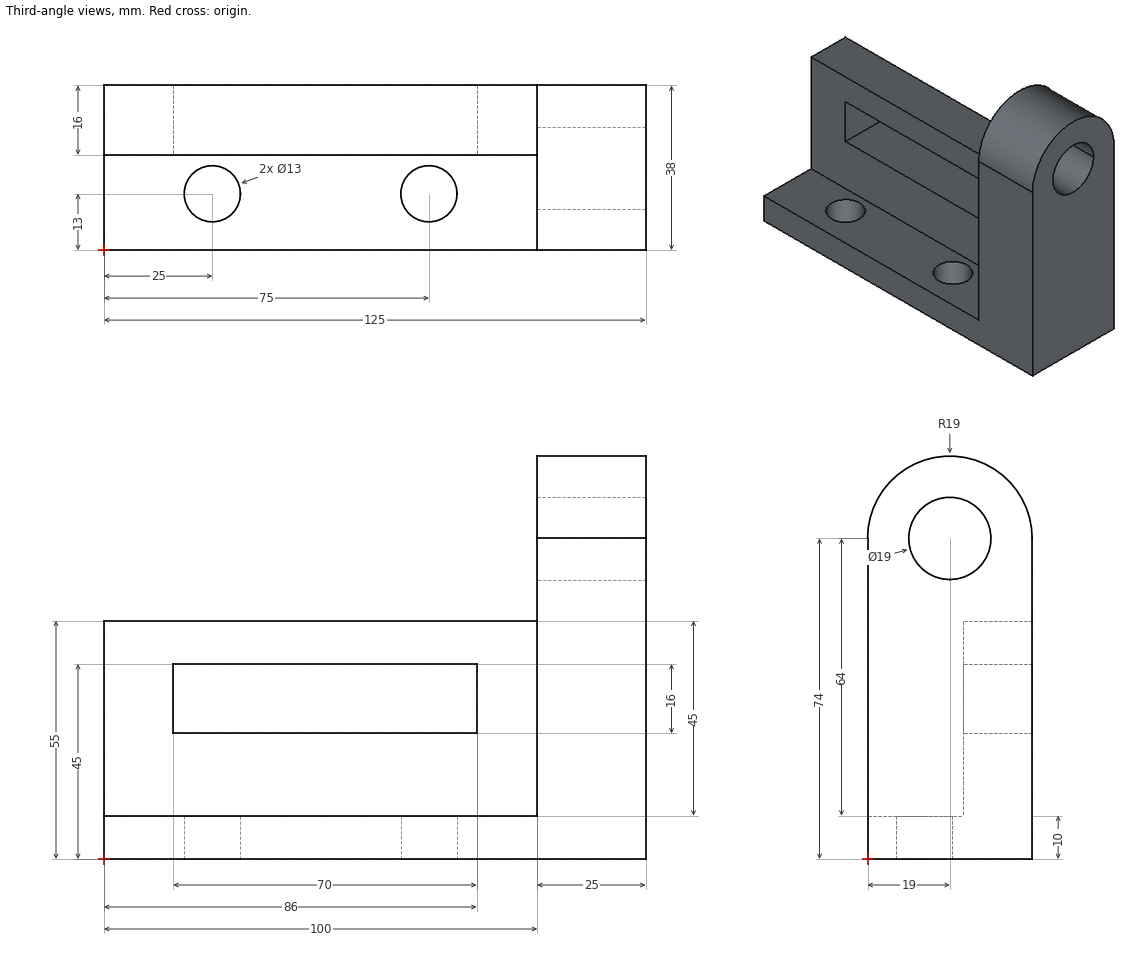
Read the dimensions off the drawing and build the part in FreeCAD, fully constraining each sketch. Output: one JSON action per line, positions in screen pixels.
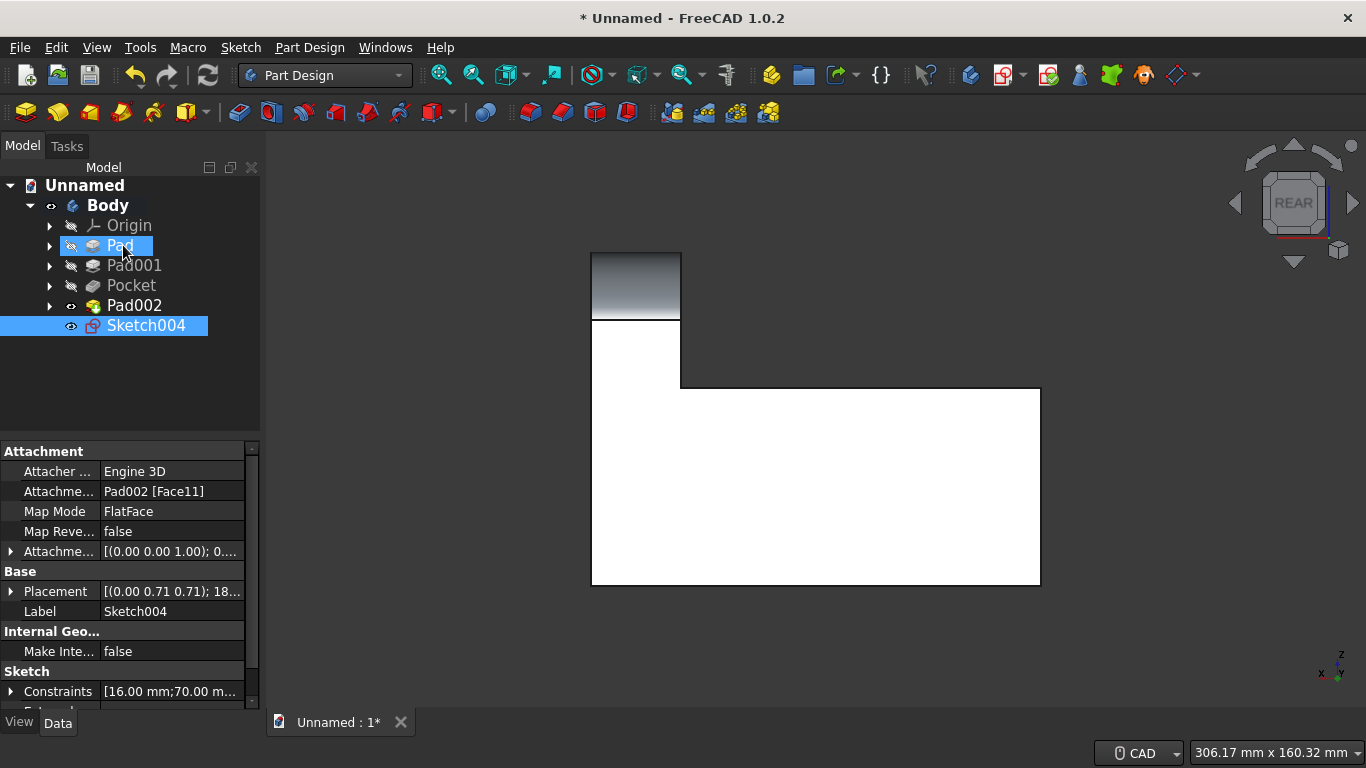
{"action": "left_click", "coordinate": [240, 112]}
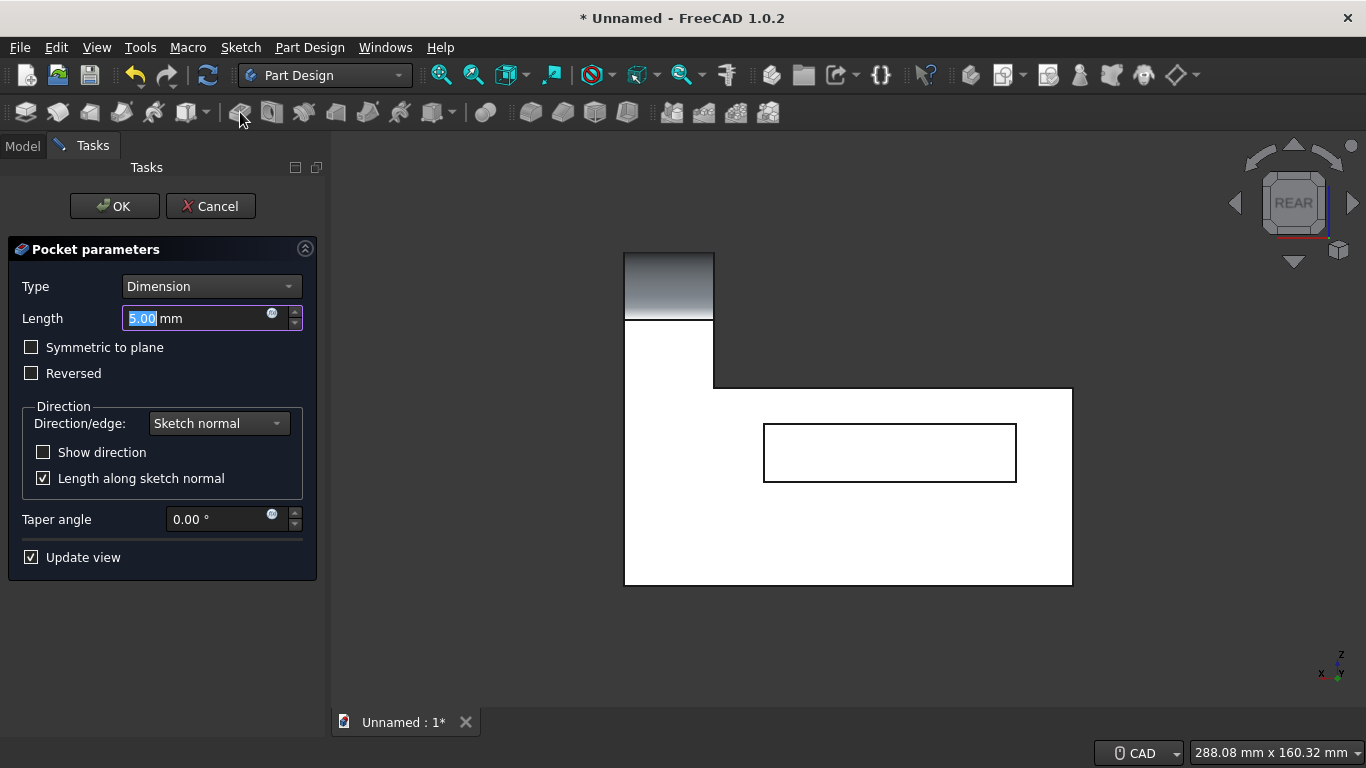
{"action": "type", "text": "16"}
{"action": "key", "text": "Tab"}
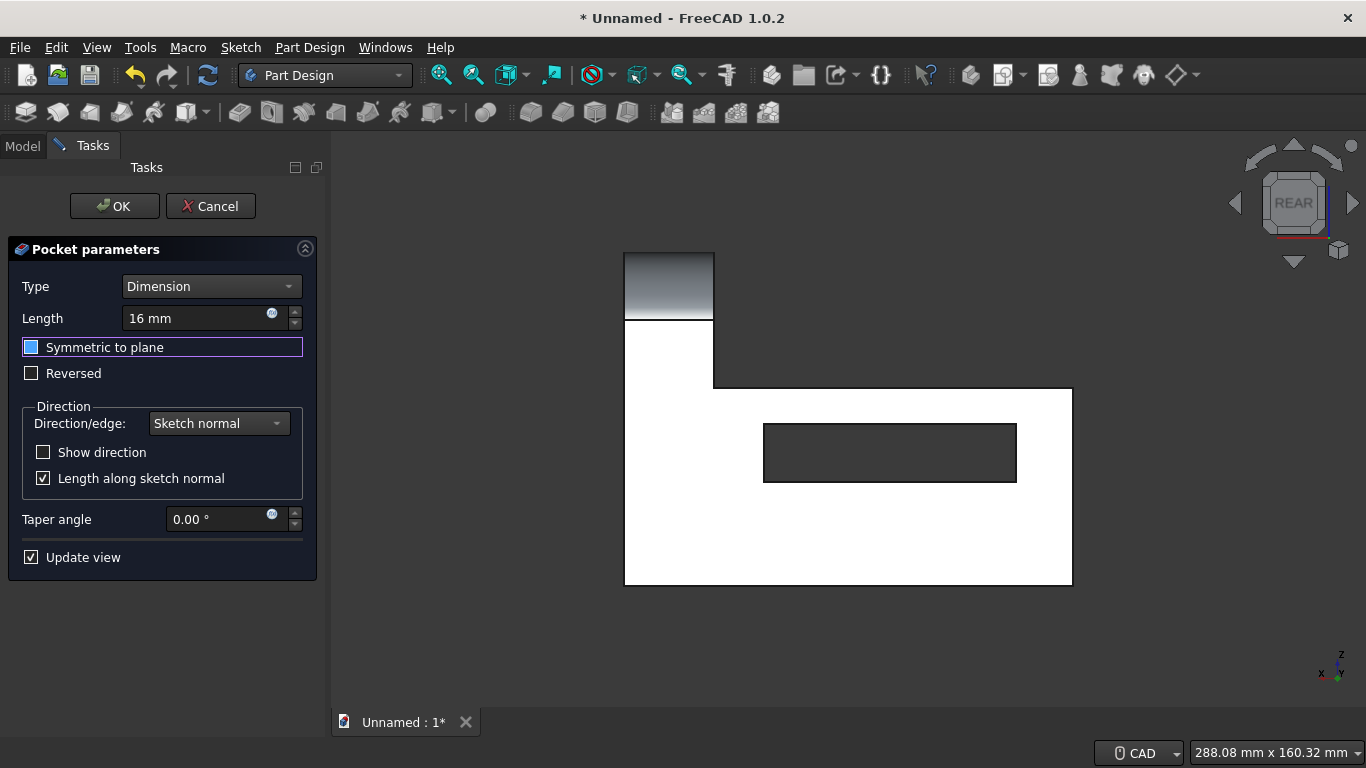
{"action": "left_click", "coordinate": [115, 206]}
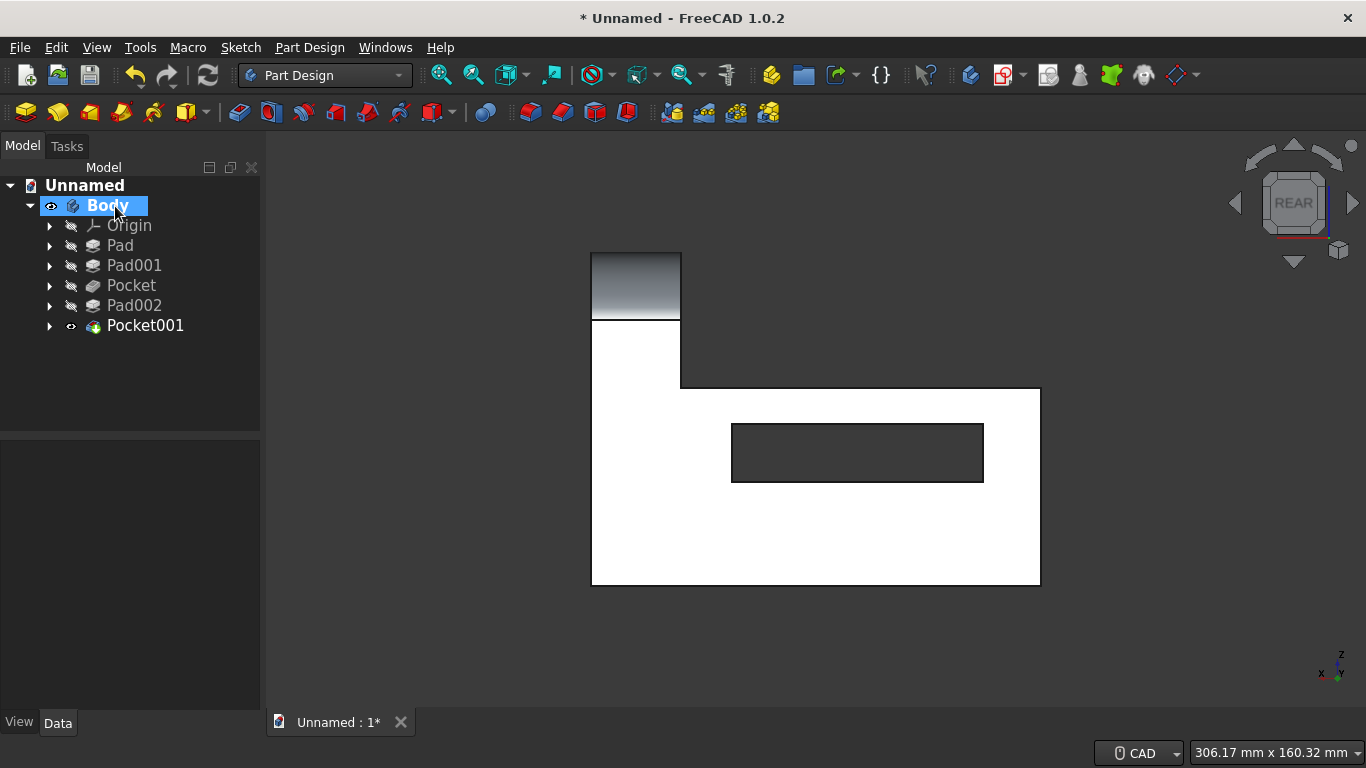
{"action": "key", "text": "0"}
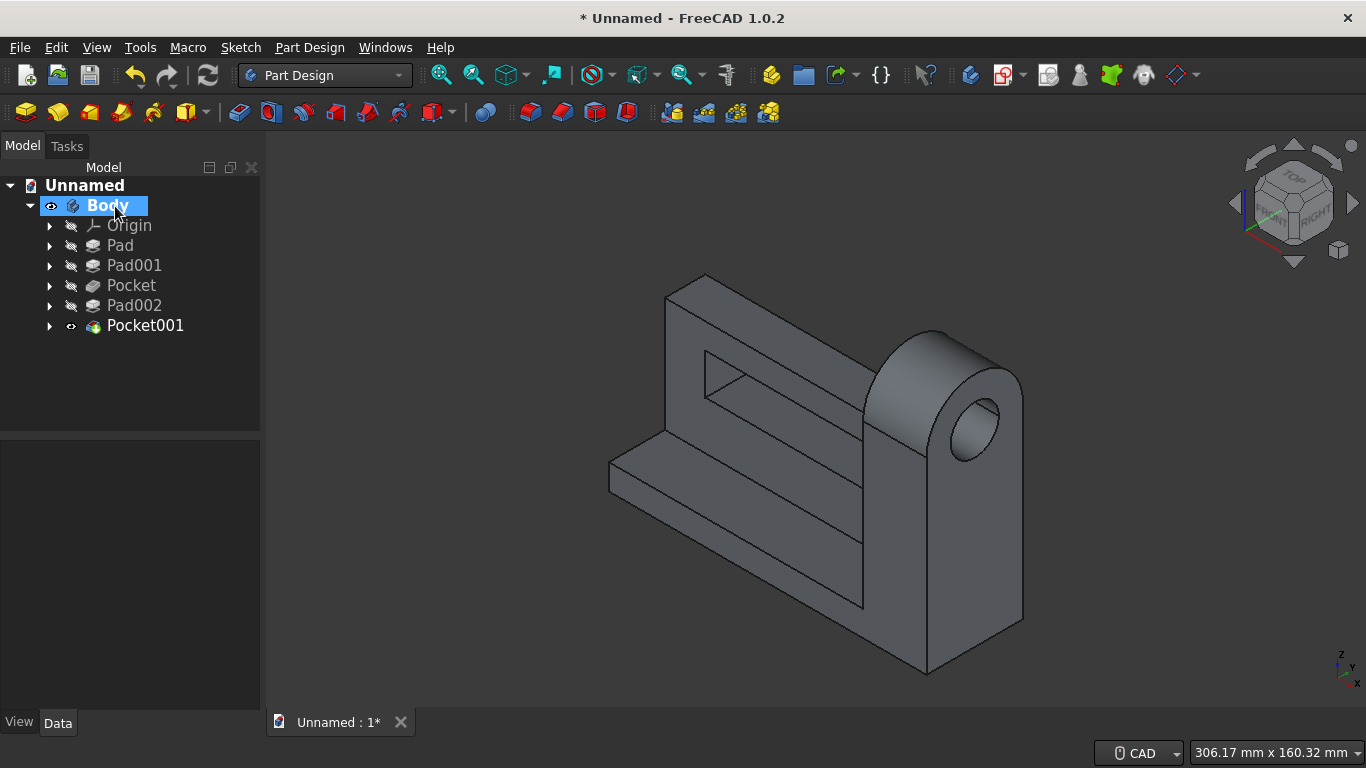
{"action": "left_click", "coordinate": [837, 560]}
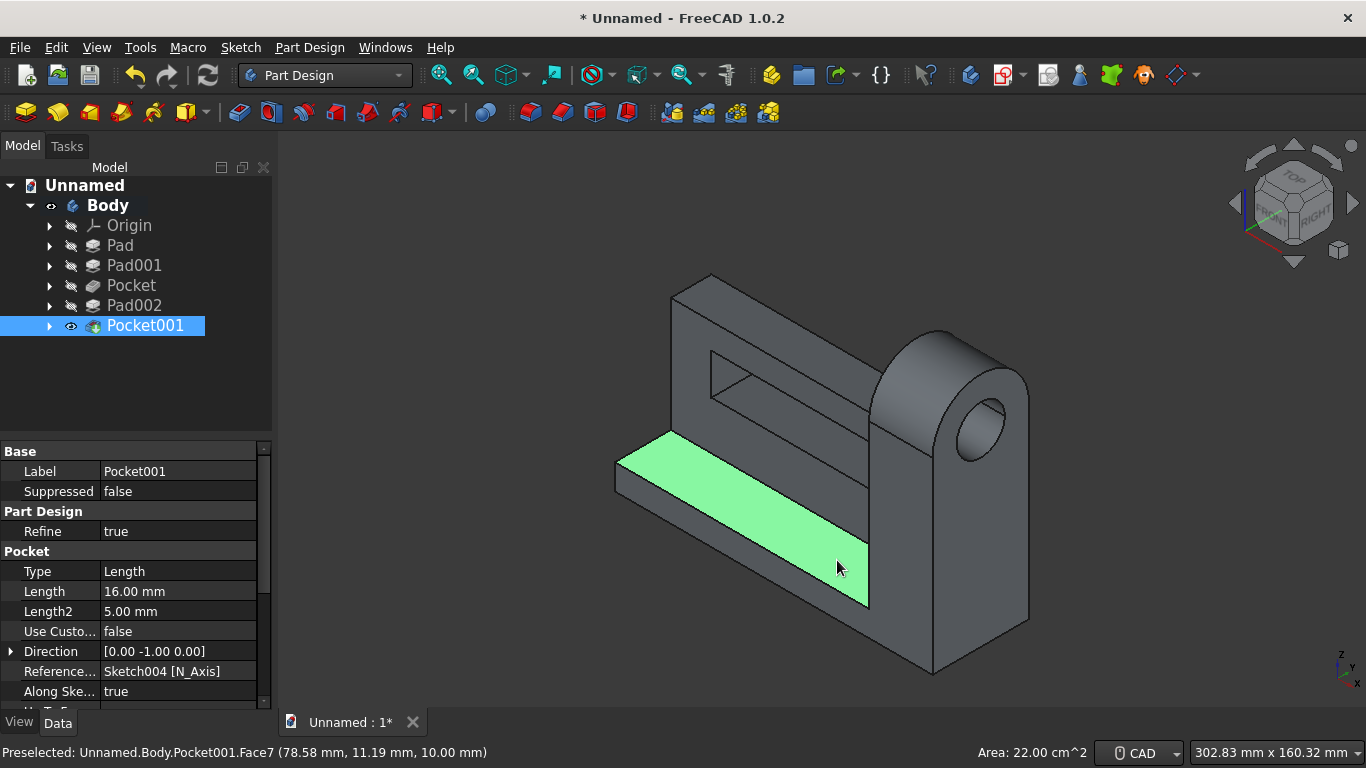
{"action": "left_click", "coordinate": [1004, 76]}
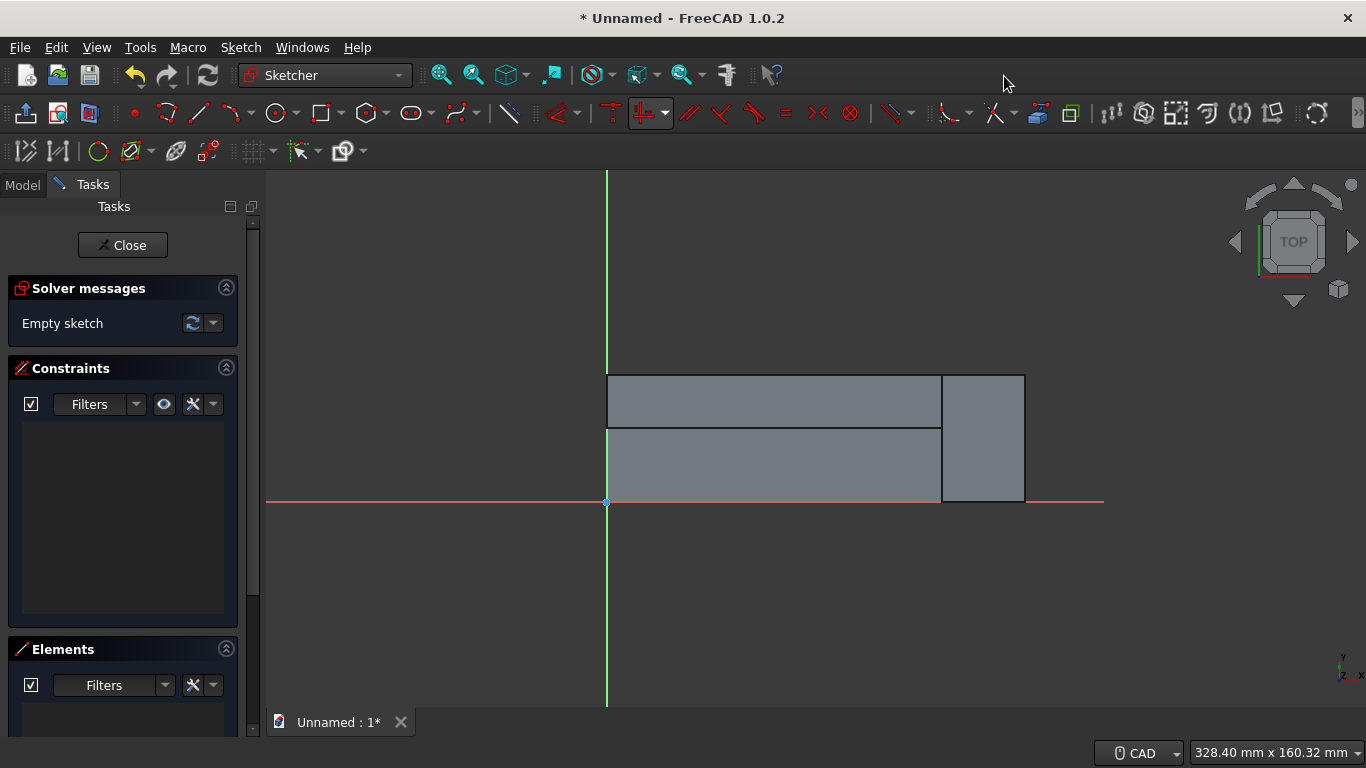
{"action": "left_click", "coordinate": [90, 114]}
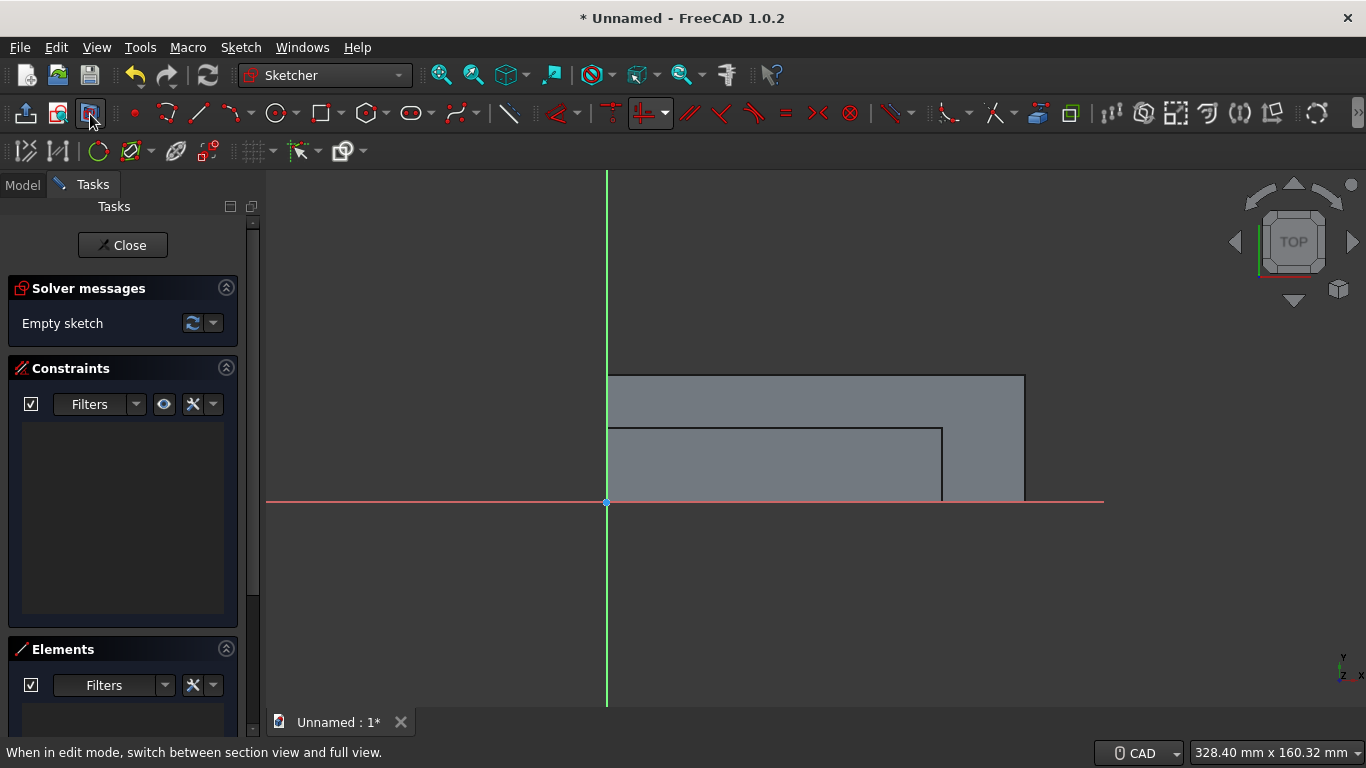
{"action": "scroll", "coordinate": [740, 495], "scroll_direction": "up", "scroll_amount": 4}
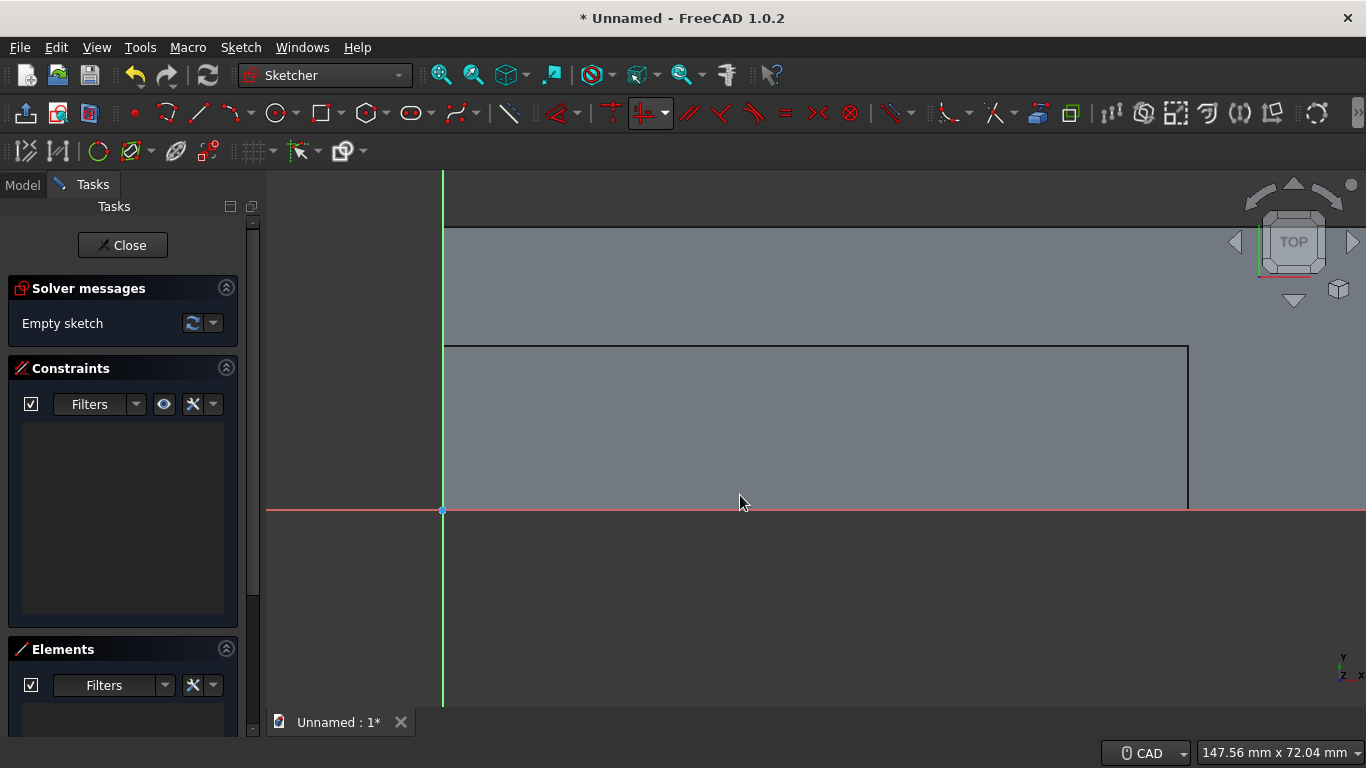
{"action": "left_click", "coordinate": [276, 114]}